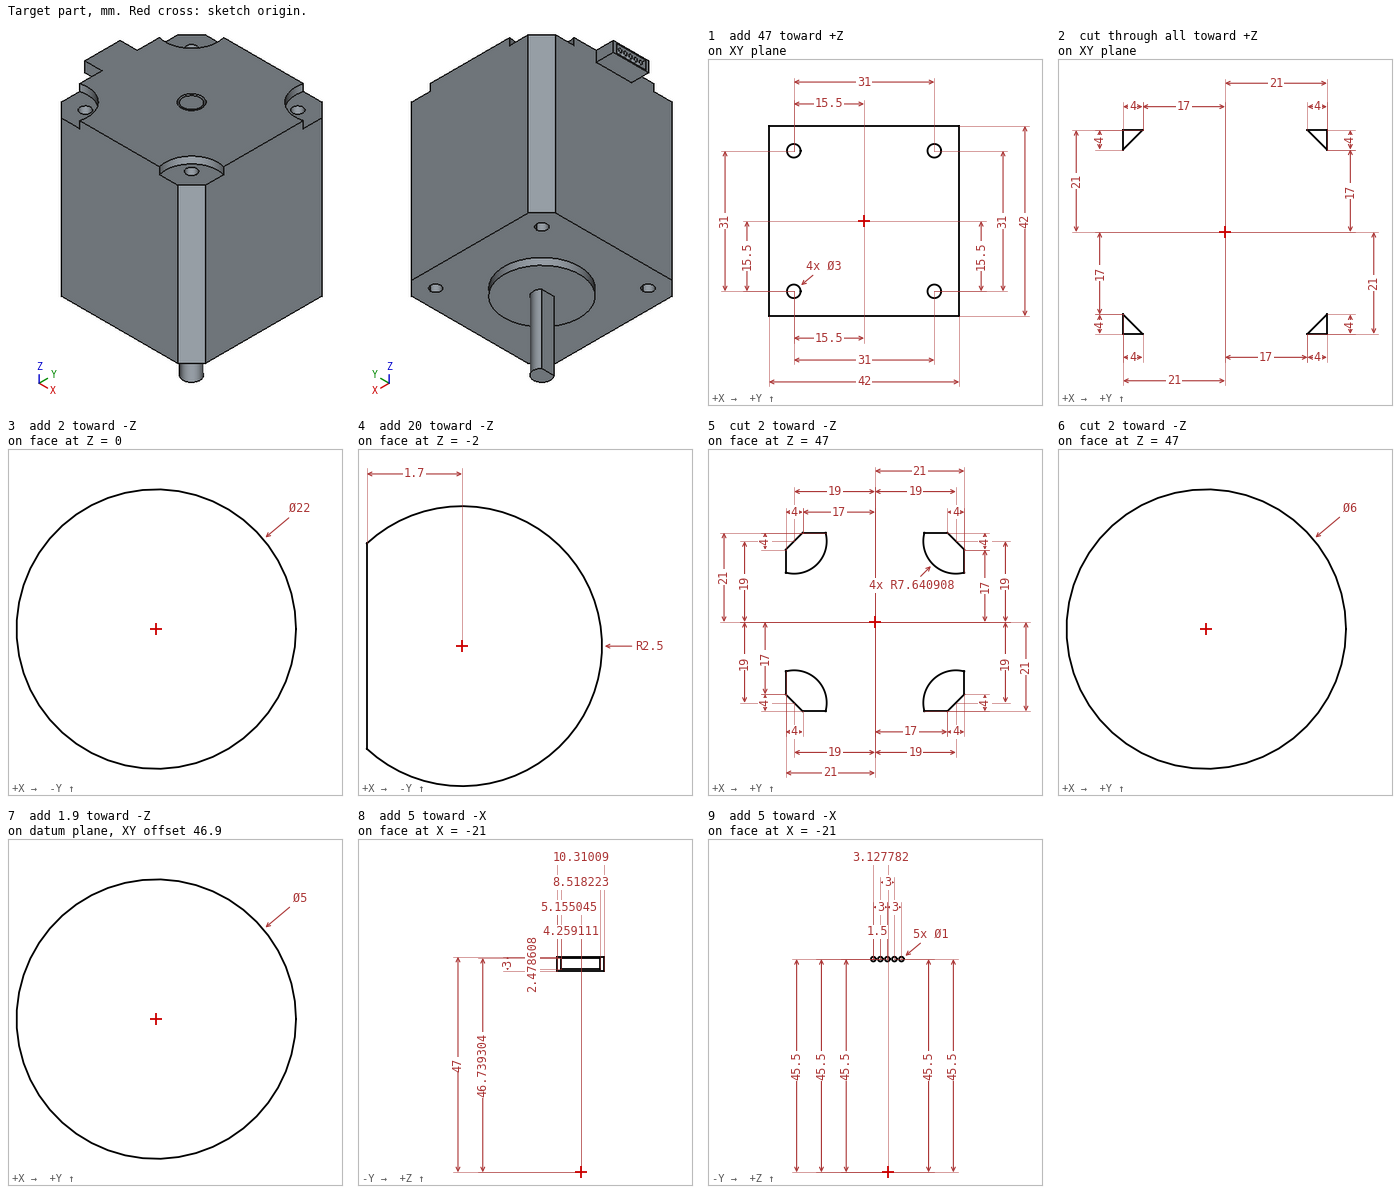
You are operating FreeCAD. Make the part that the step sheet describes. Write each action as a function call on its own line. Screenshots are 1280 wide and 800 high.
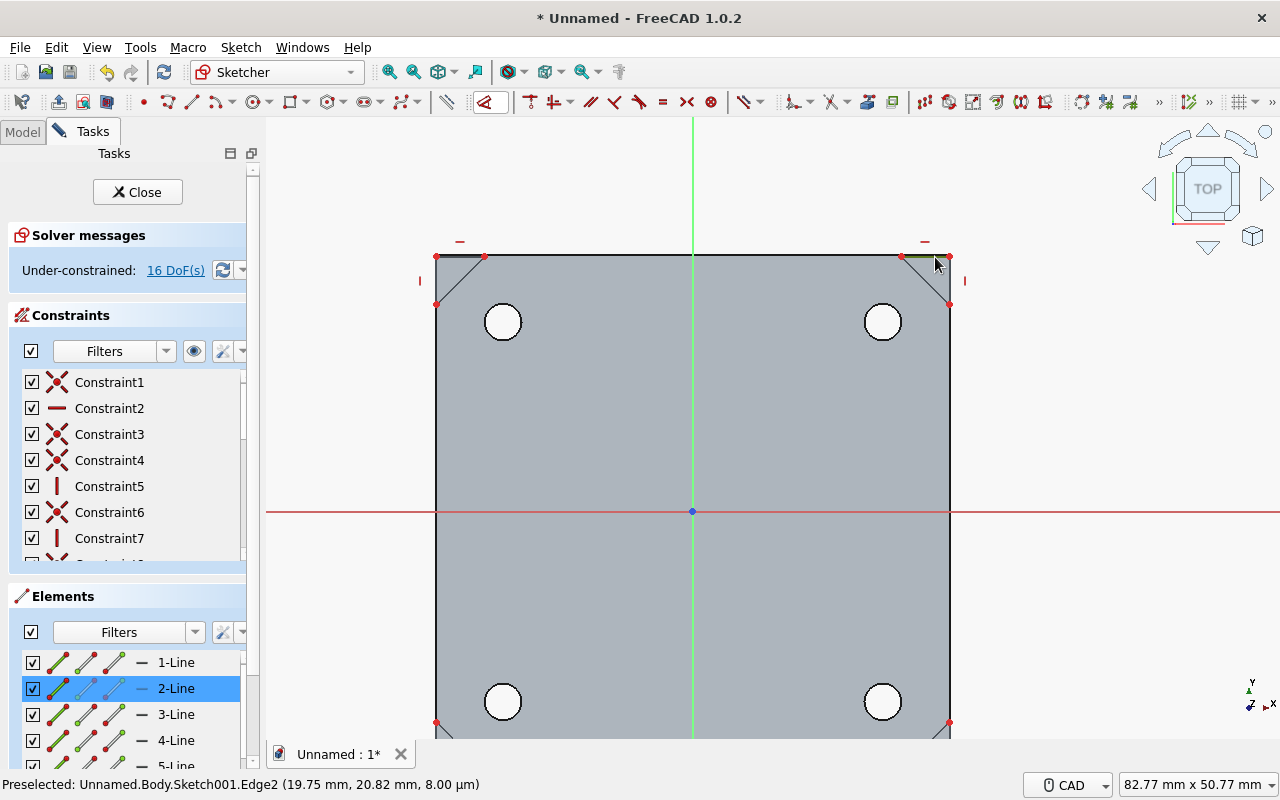
click(502, 102)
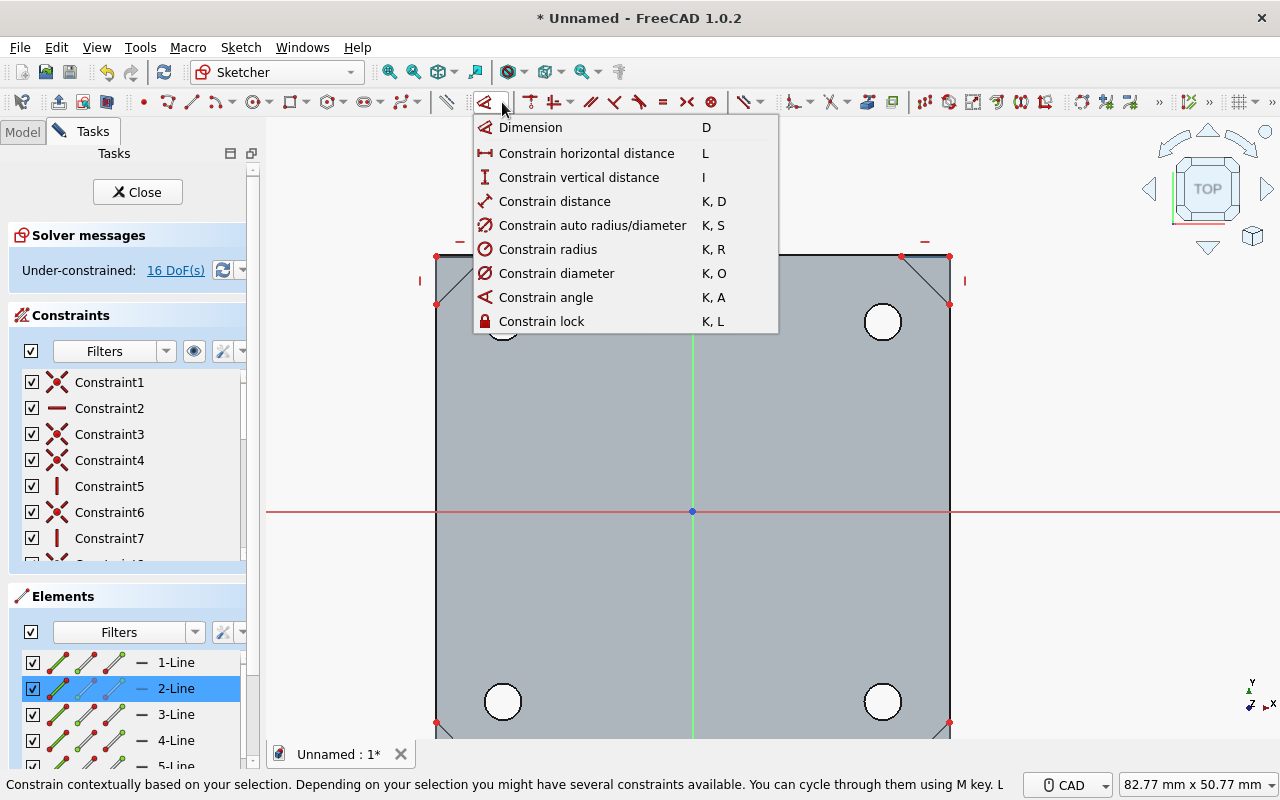
click(626, 153)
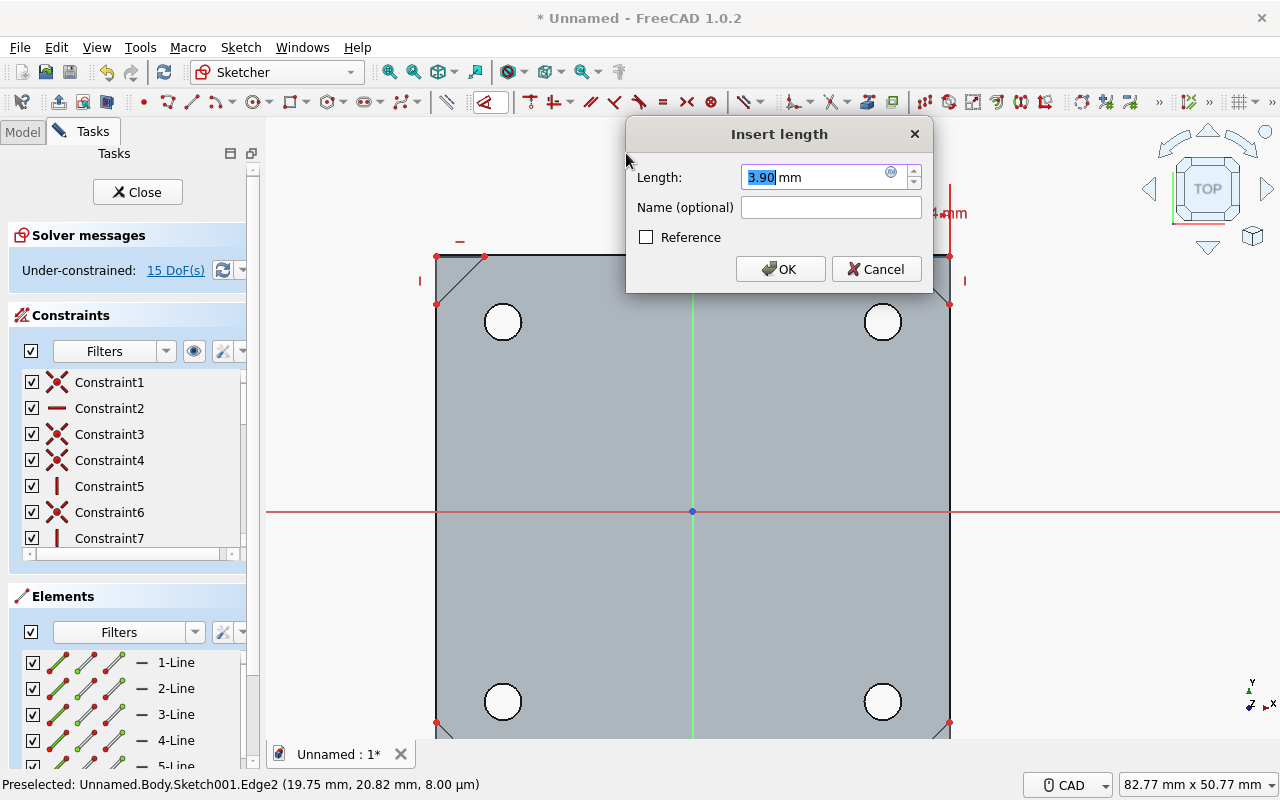
text(4)
key(Return)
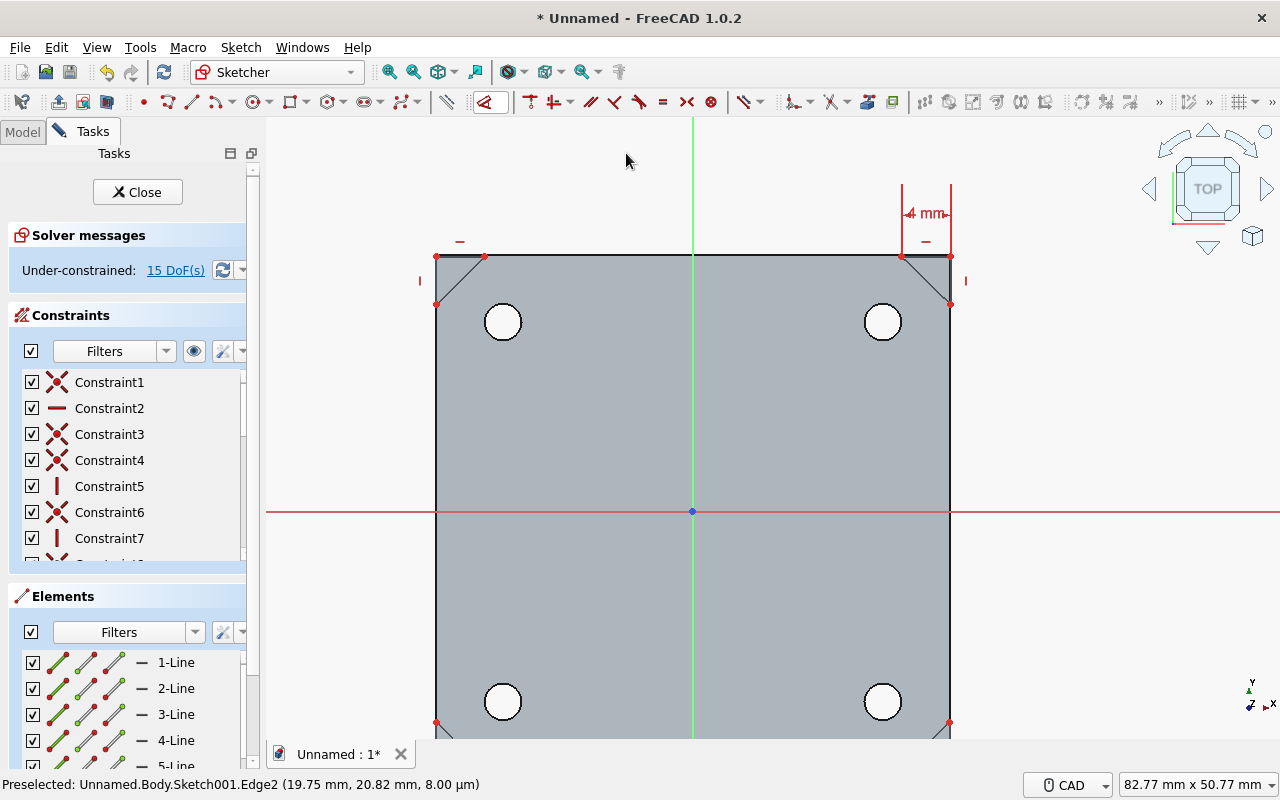
click(951, 271)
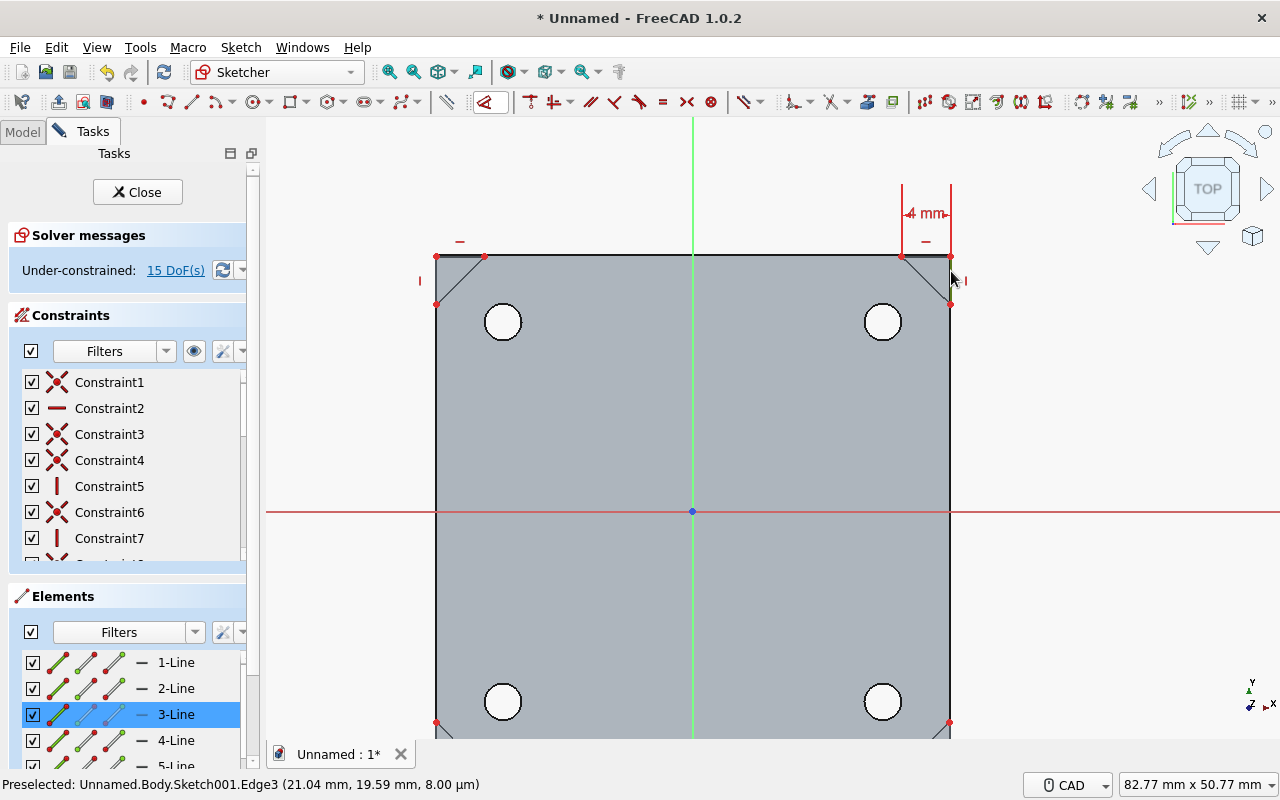
key(i)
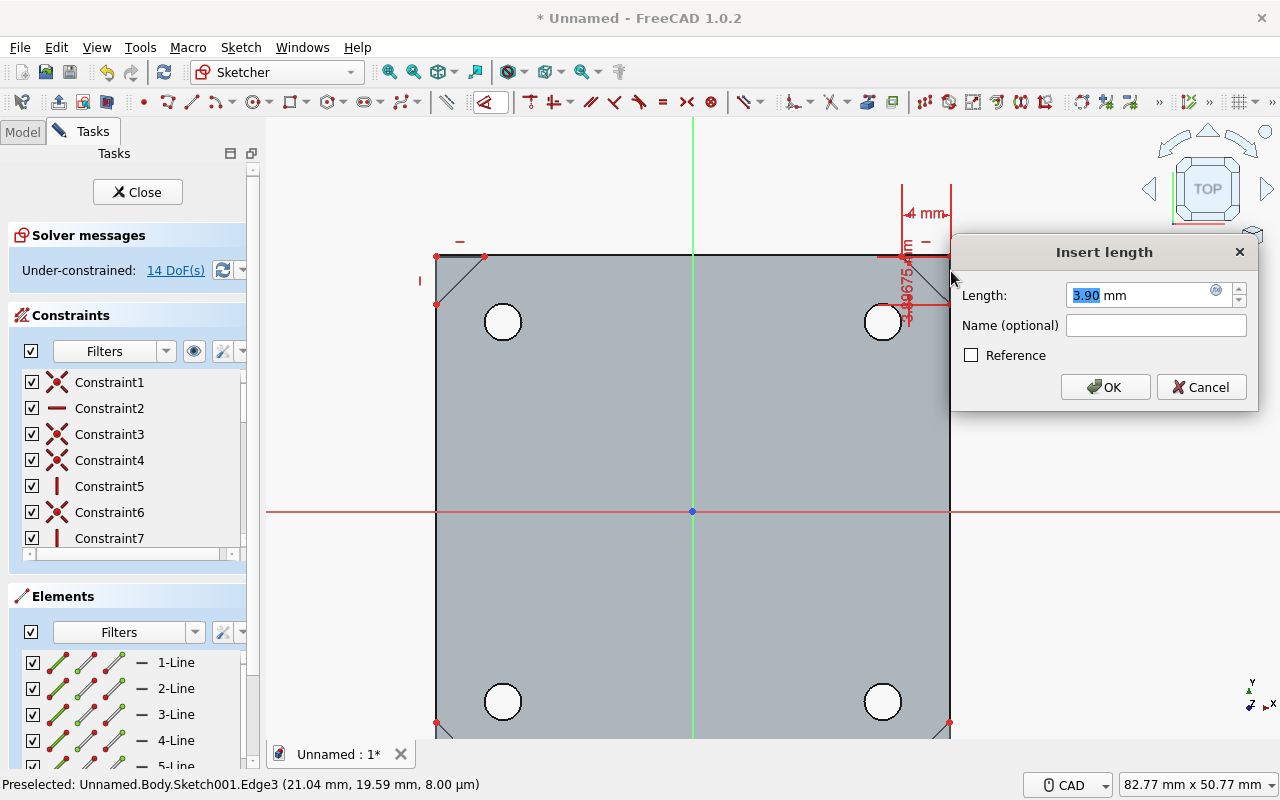
text(4)
key(Return)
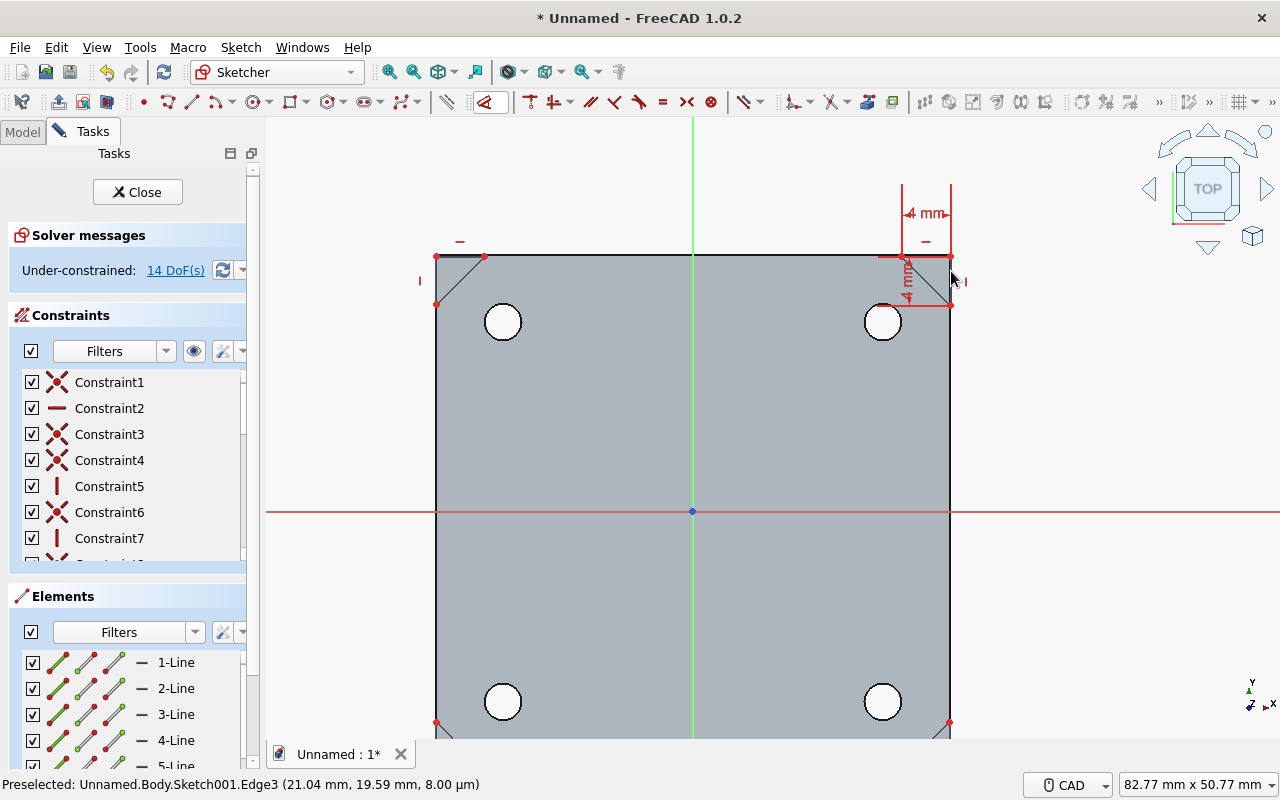
scroll(436, 290, up, 2)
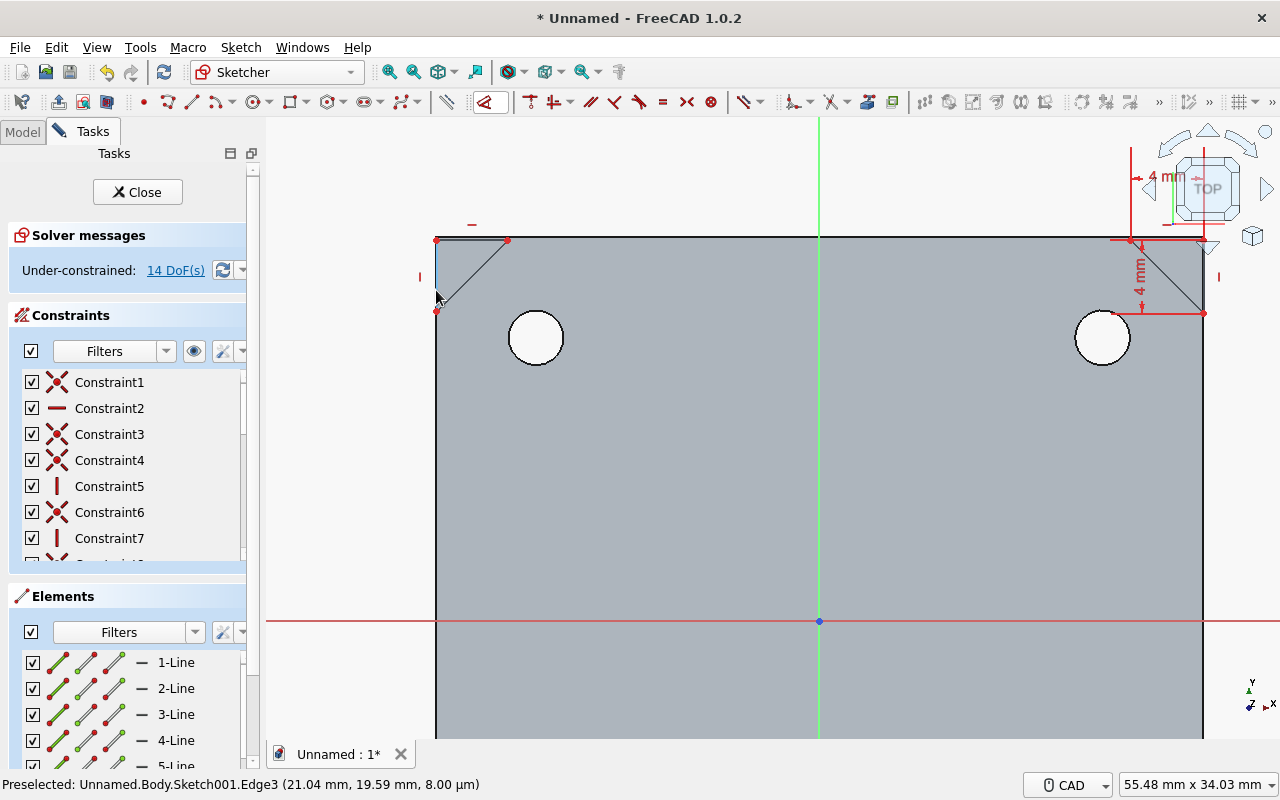
click(437, 290)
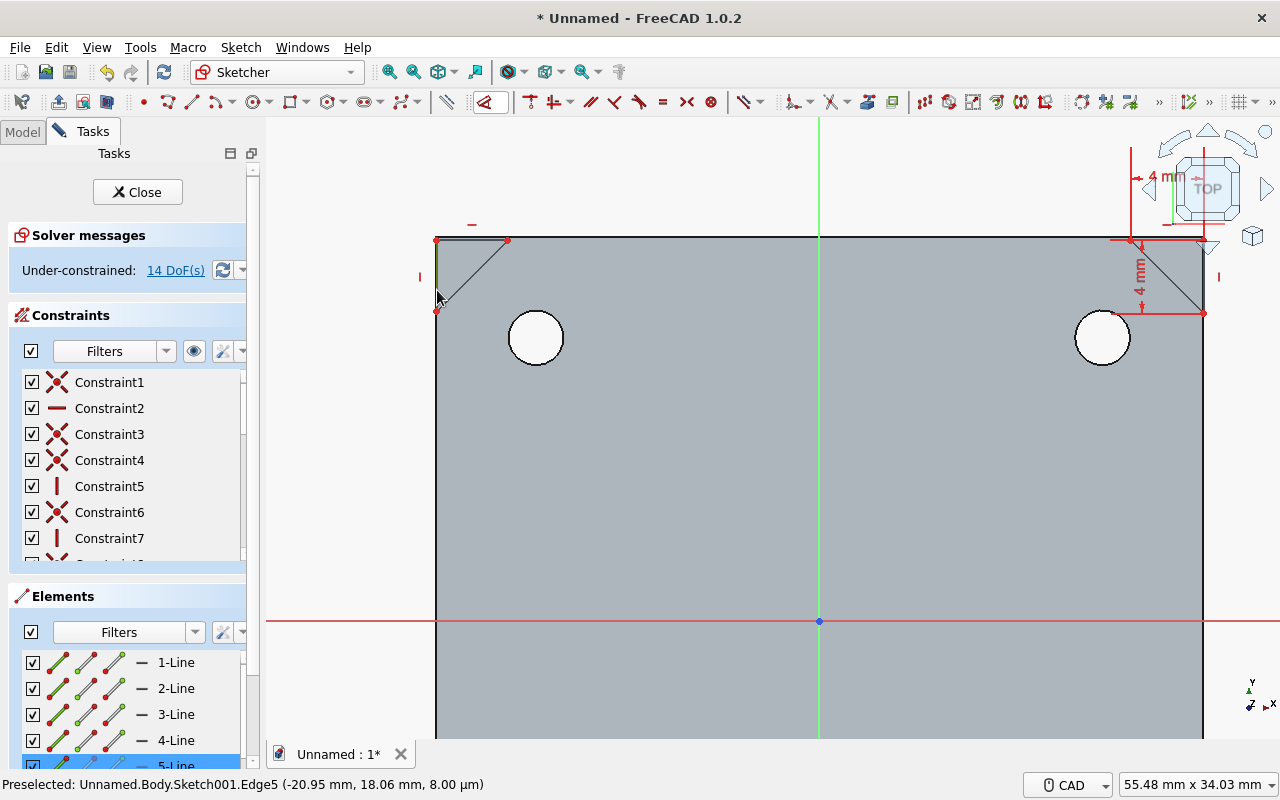
key(i)